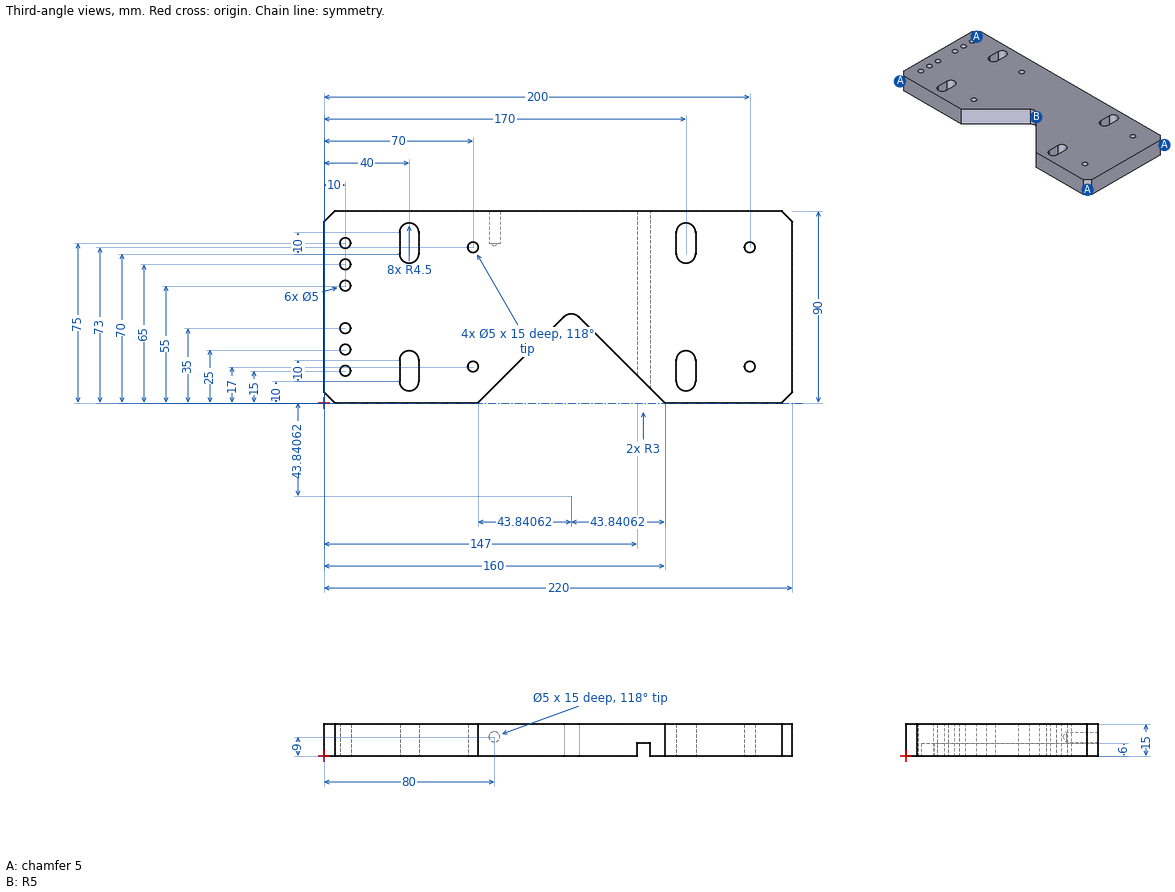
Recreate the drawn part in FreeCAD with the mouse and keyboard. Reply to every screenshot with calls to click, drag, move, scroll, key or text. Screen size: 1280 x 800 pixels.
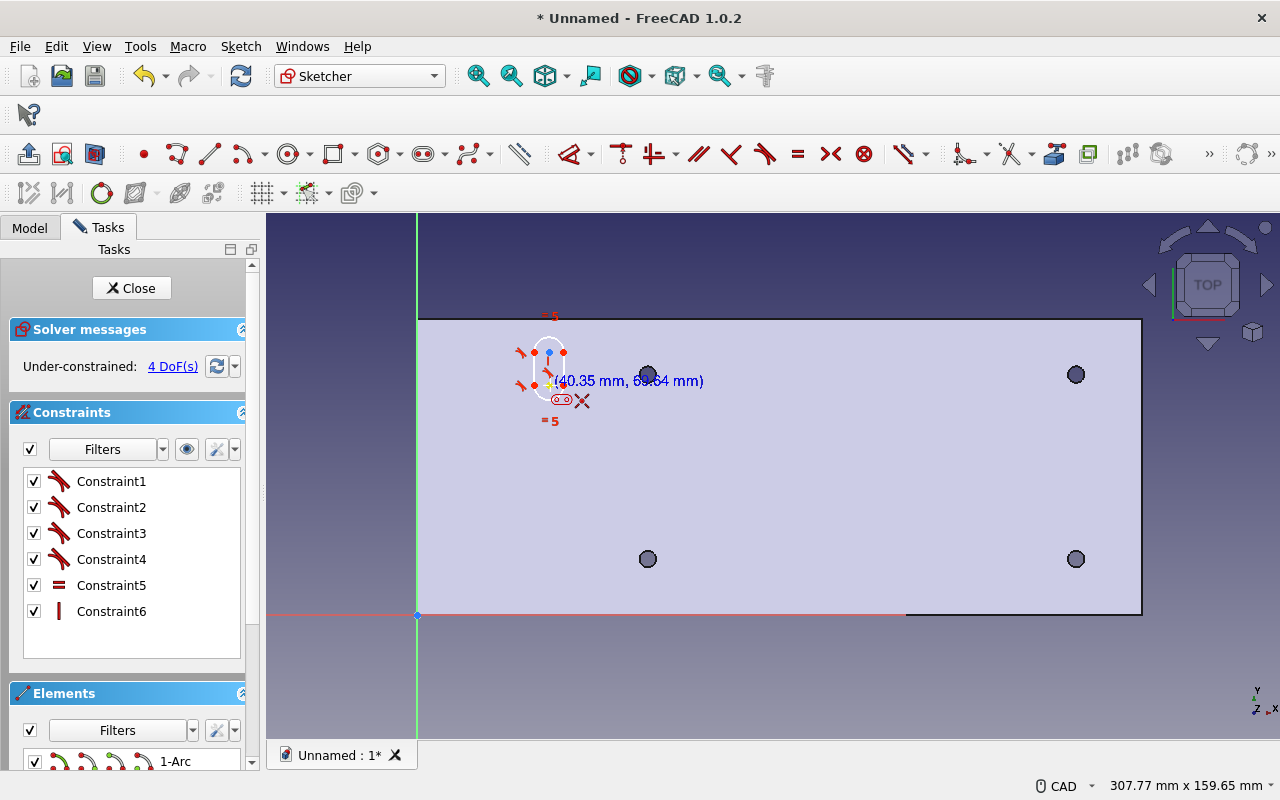
scroll(549, 582, up, 3)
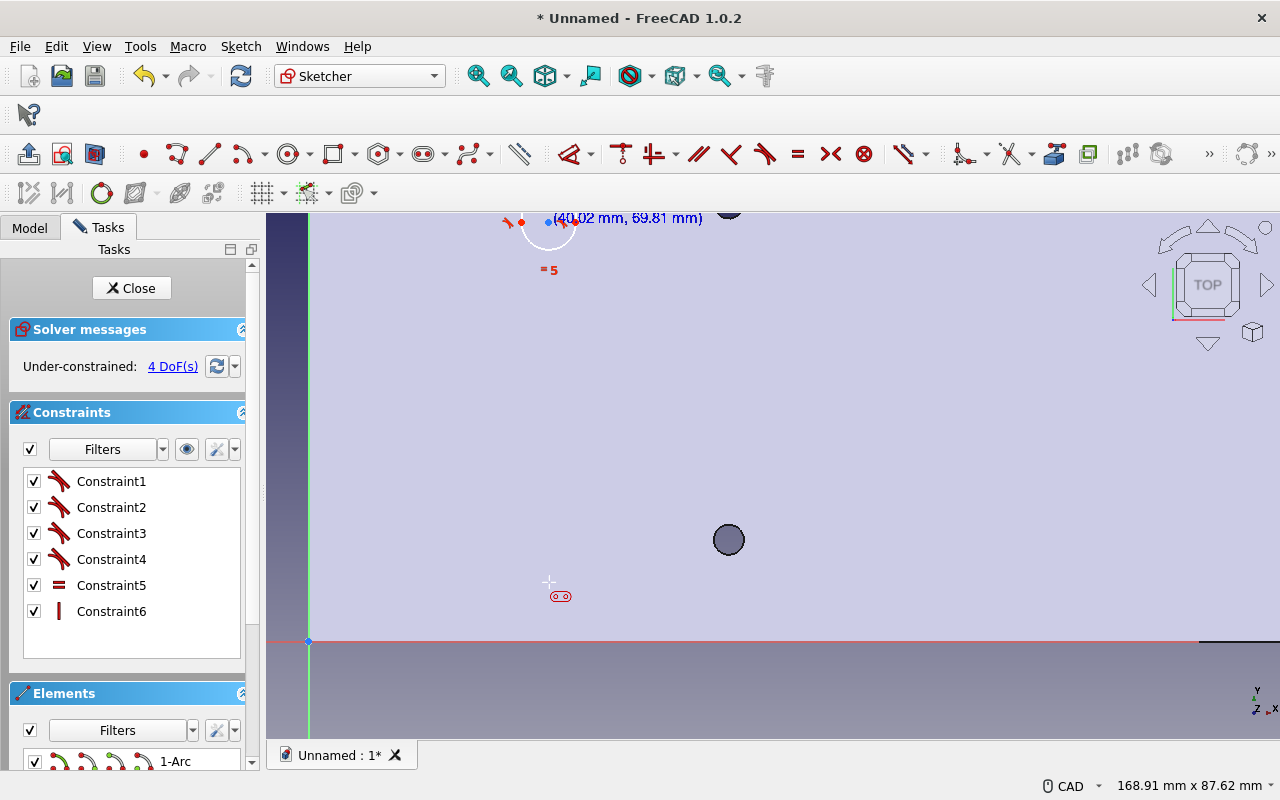
click(549, 582)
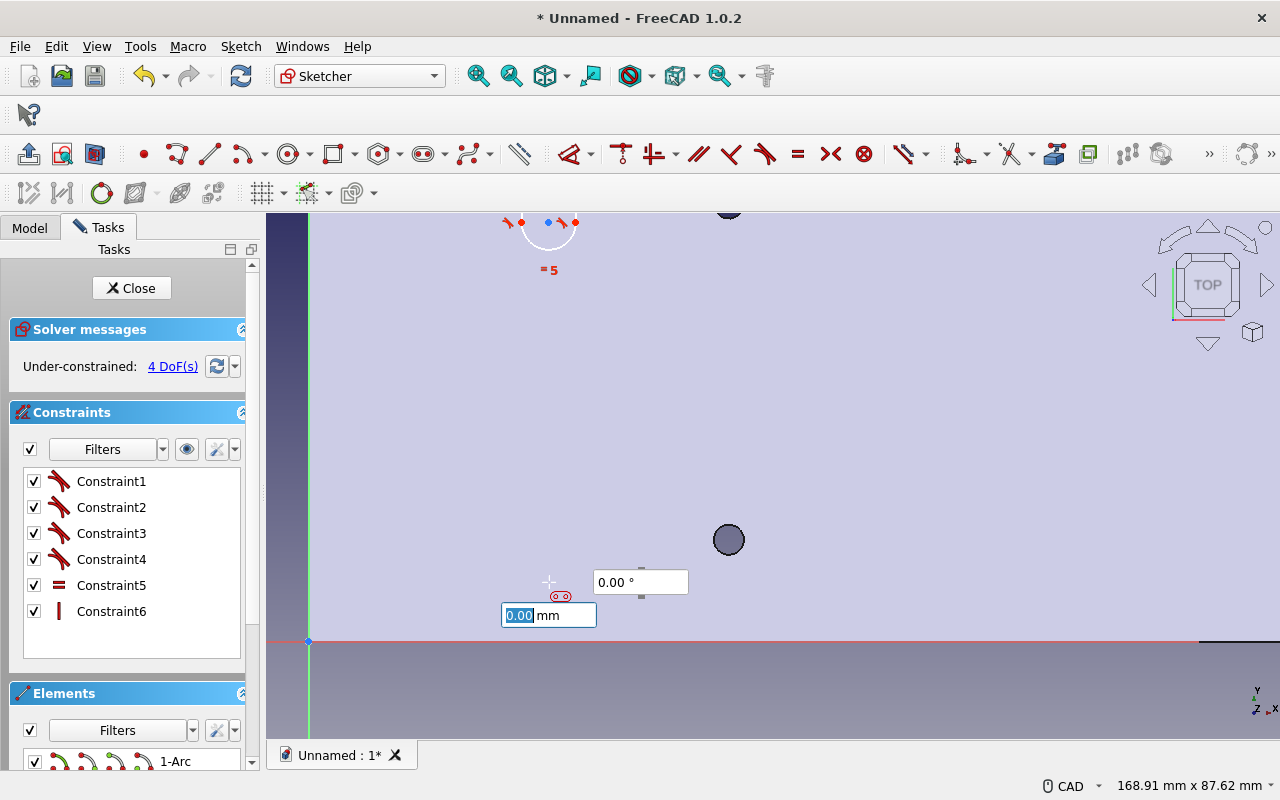
click(549, 522)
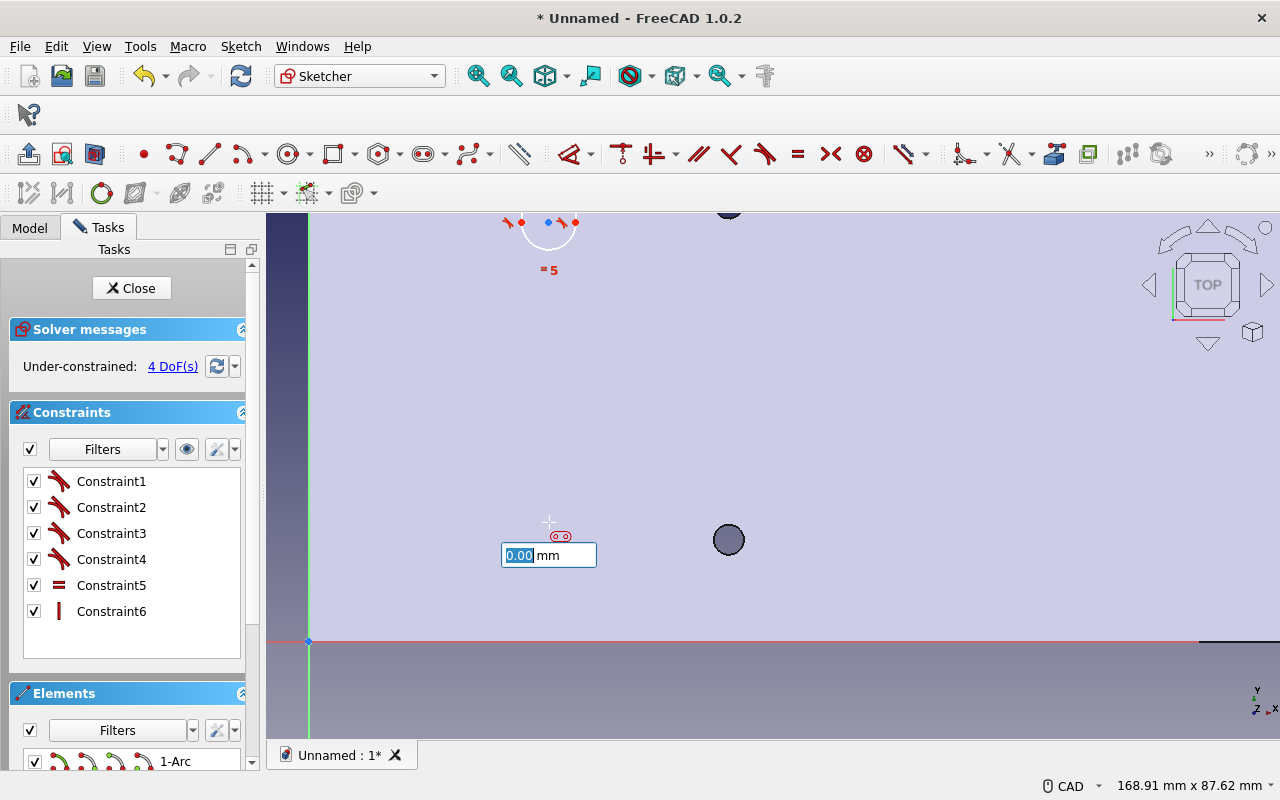
click(576, 552)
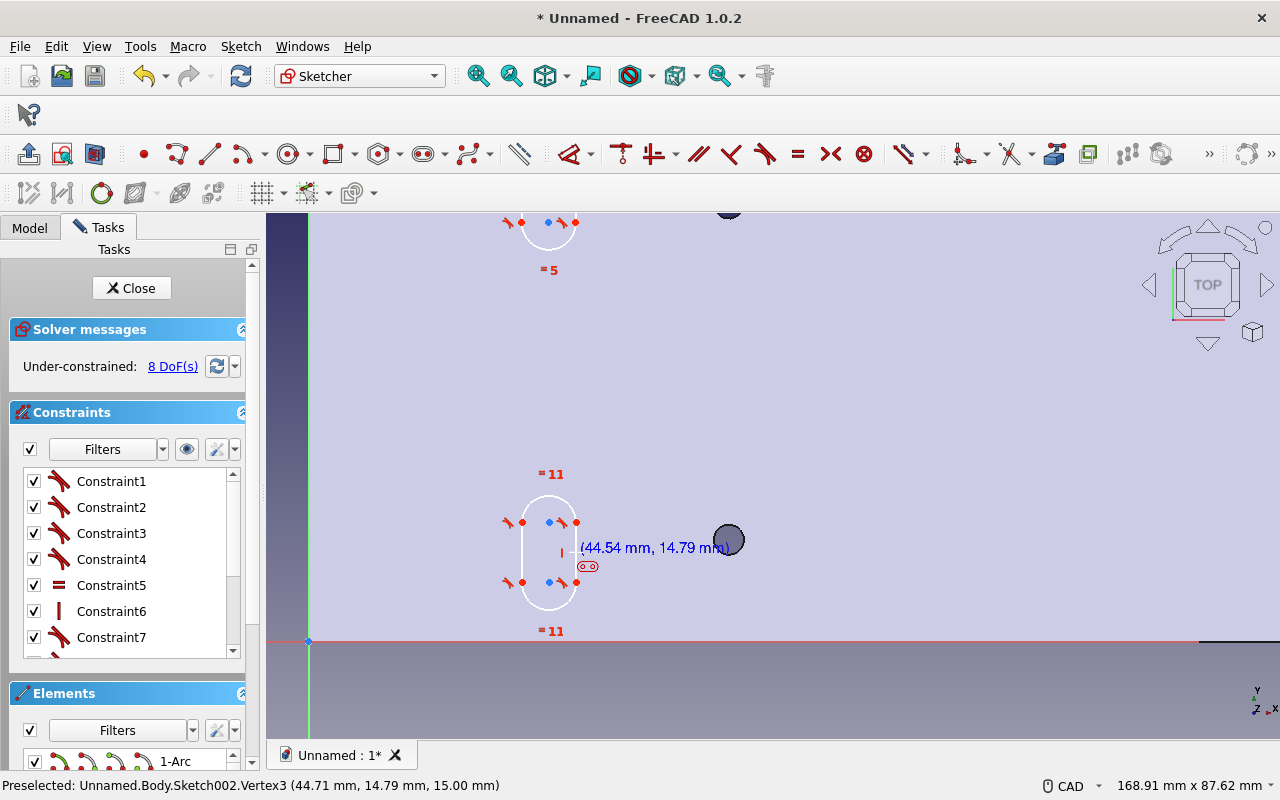
scroll(549, 583, down, 3)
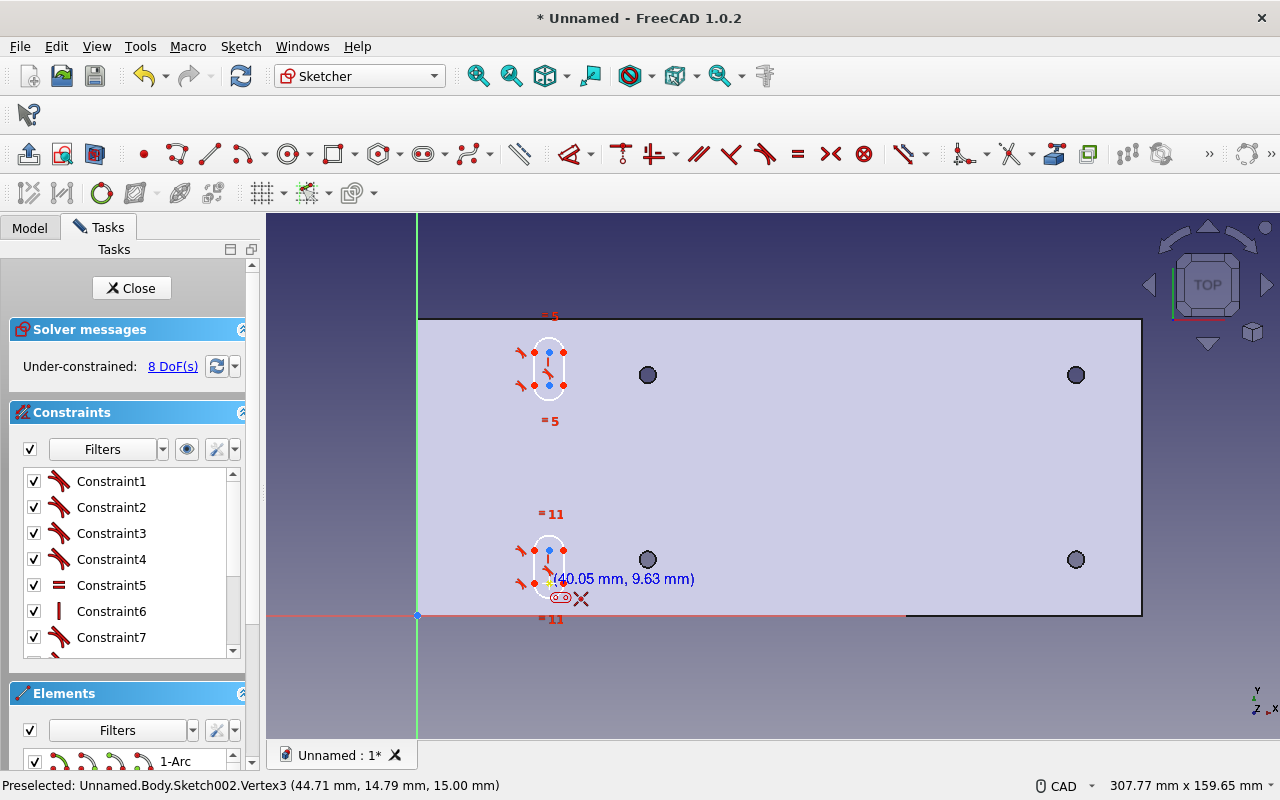
scroll(977, 385, up, 3)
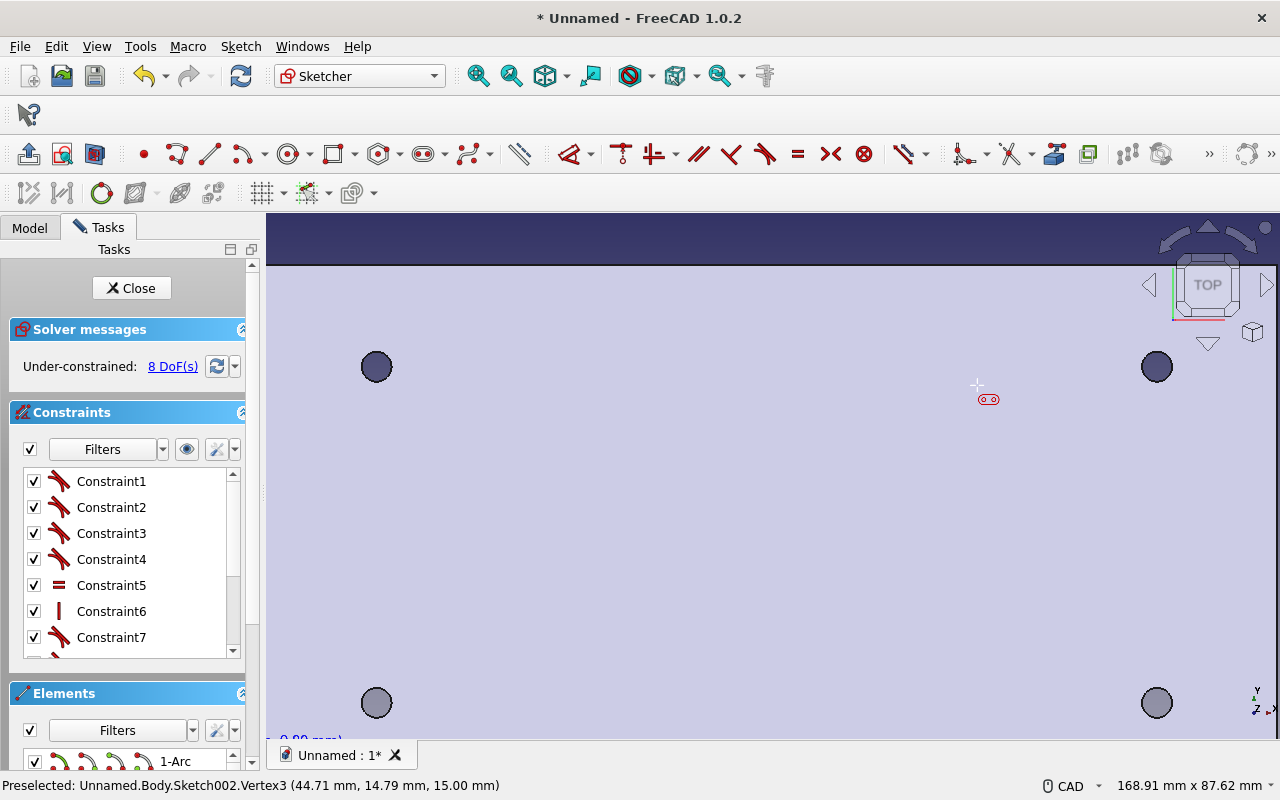
click(977, 385)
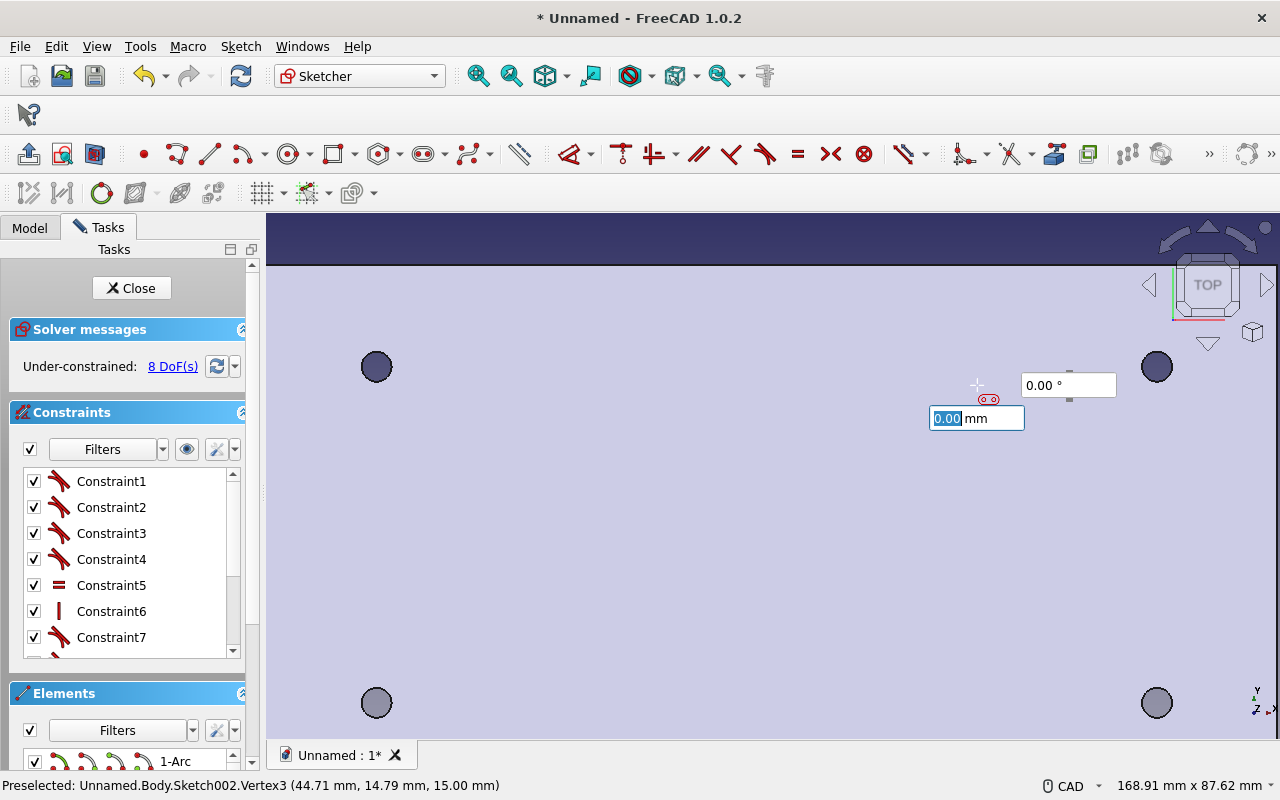
click(977, 325)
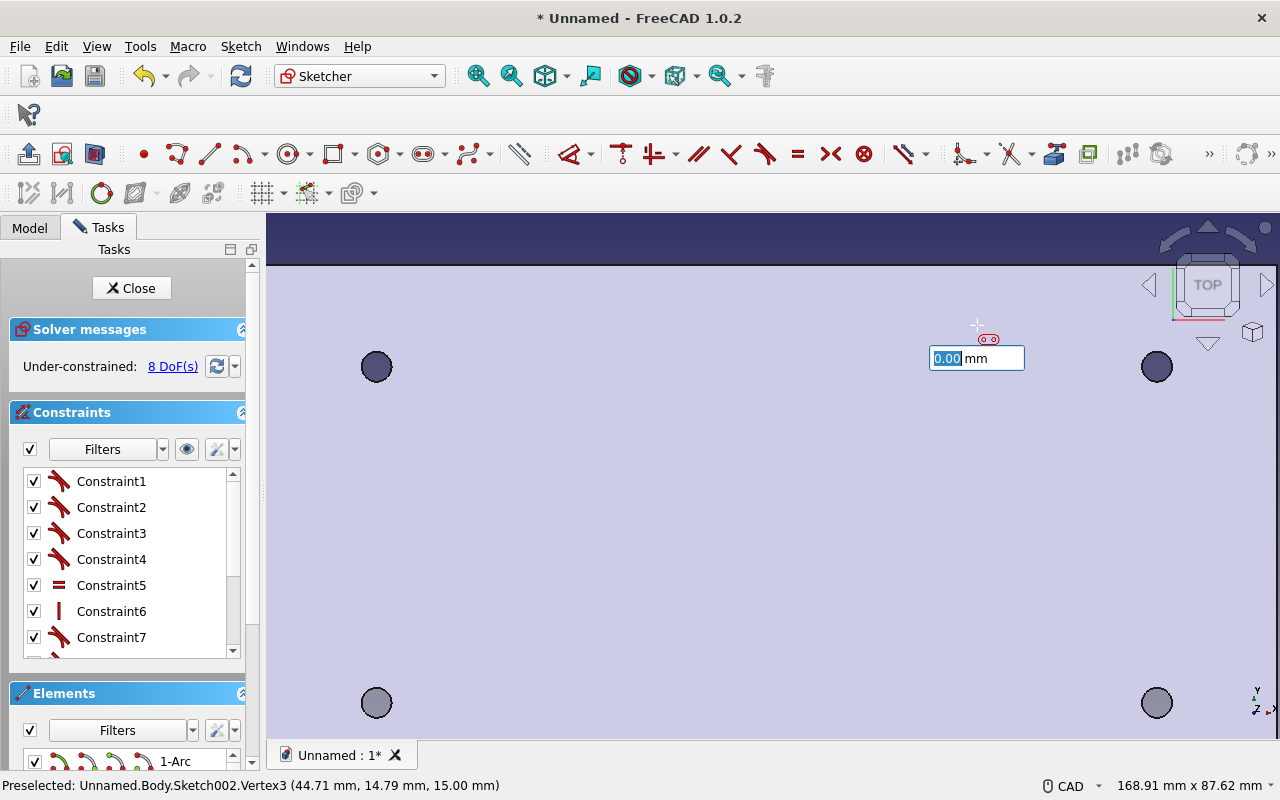
click(1004, 355)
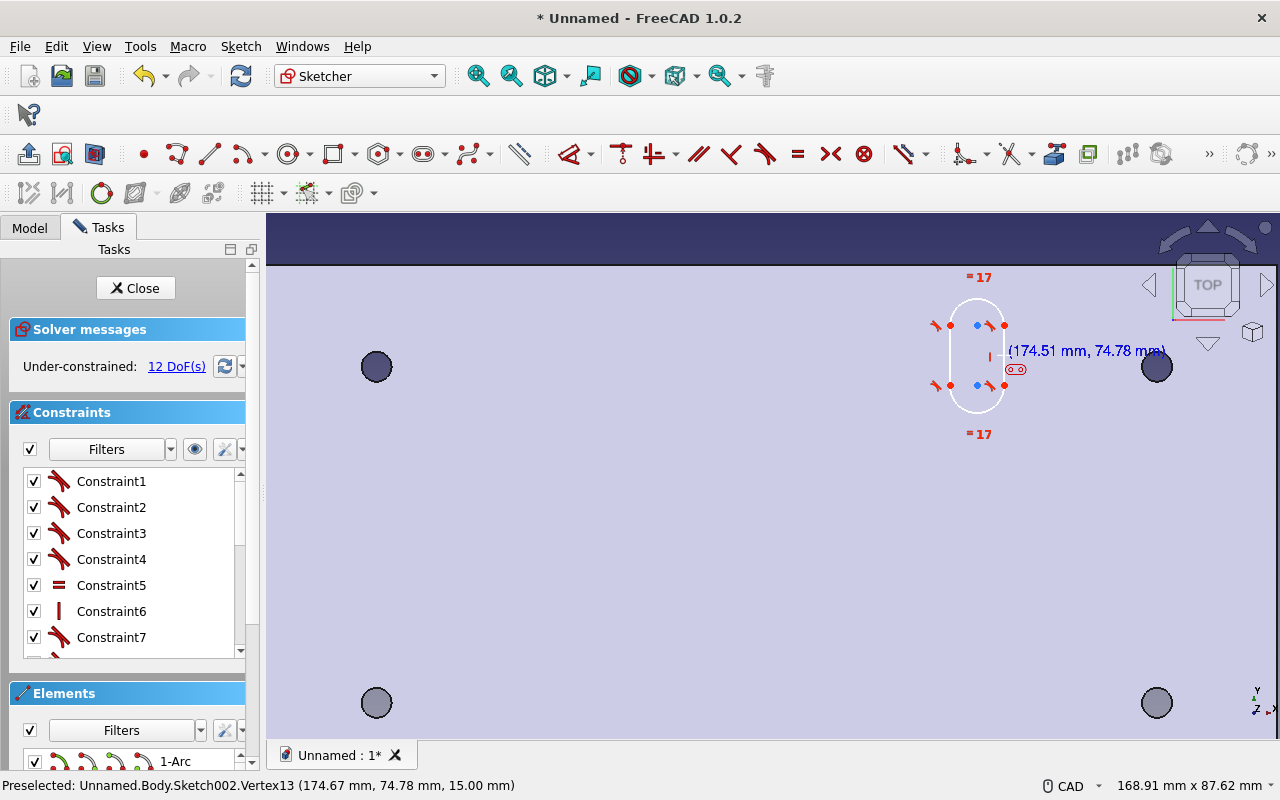
scroll(977, 384, down, 3)